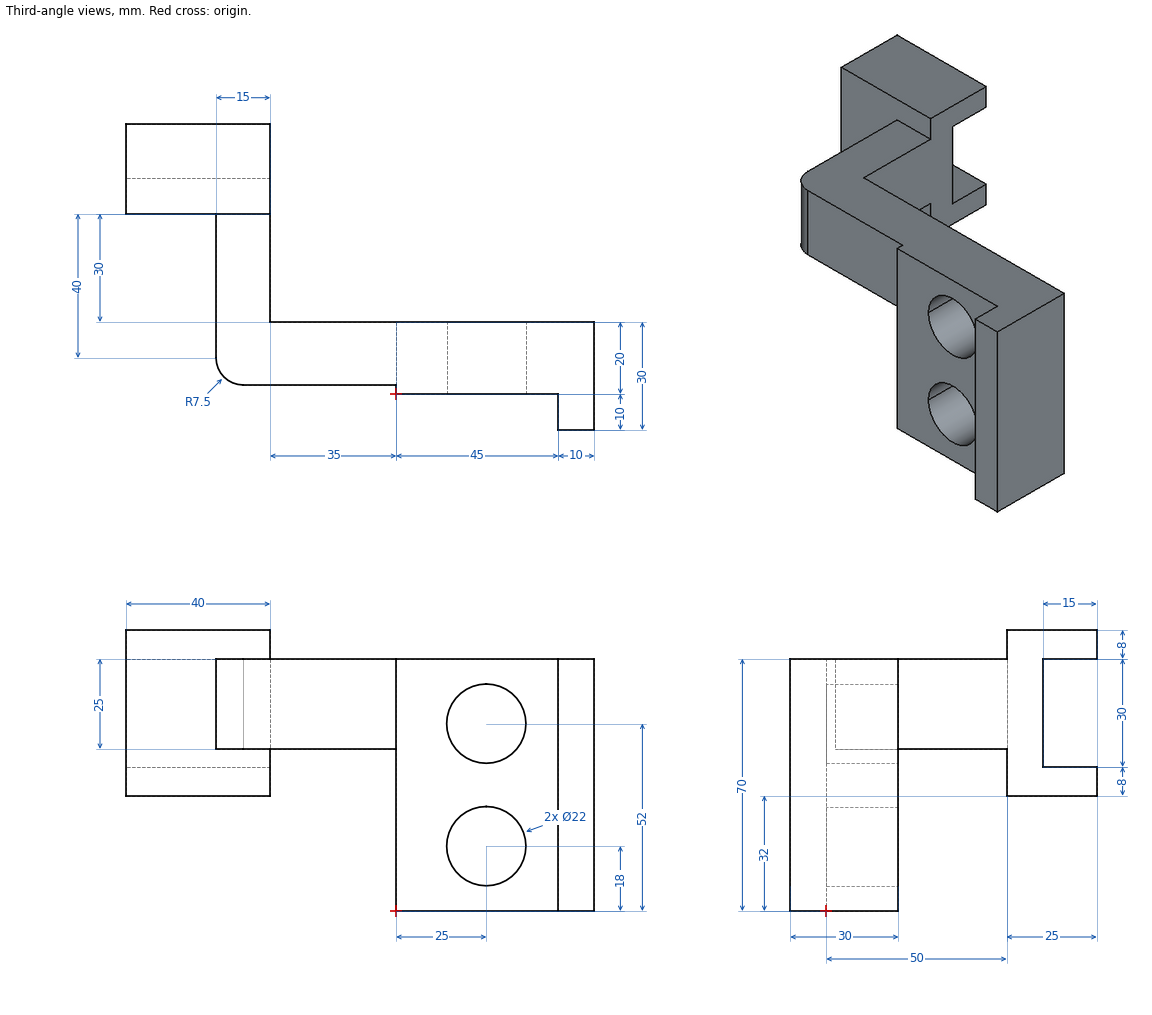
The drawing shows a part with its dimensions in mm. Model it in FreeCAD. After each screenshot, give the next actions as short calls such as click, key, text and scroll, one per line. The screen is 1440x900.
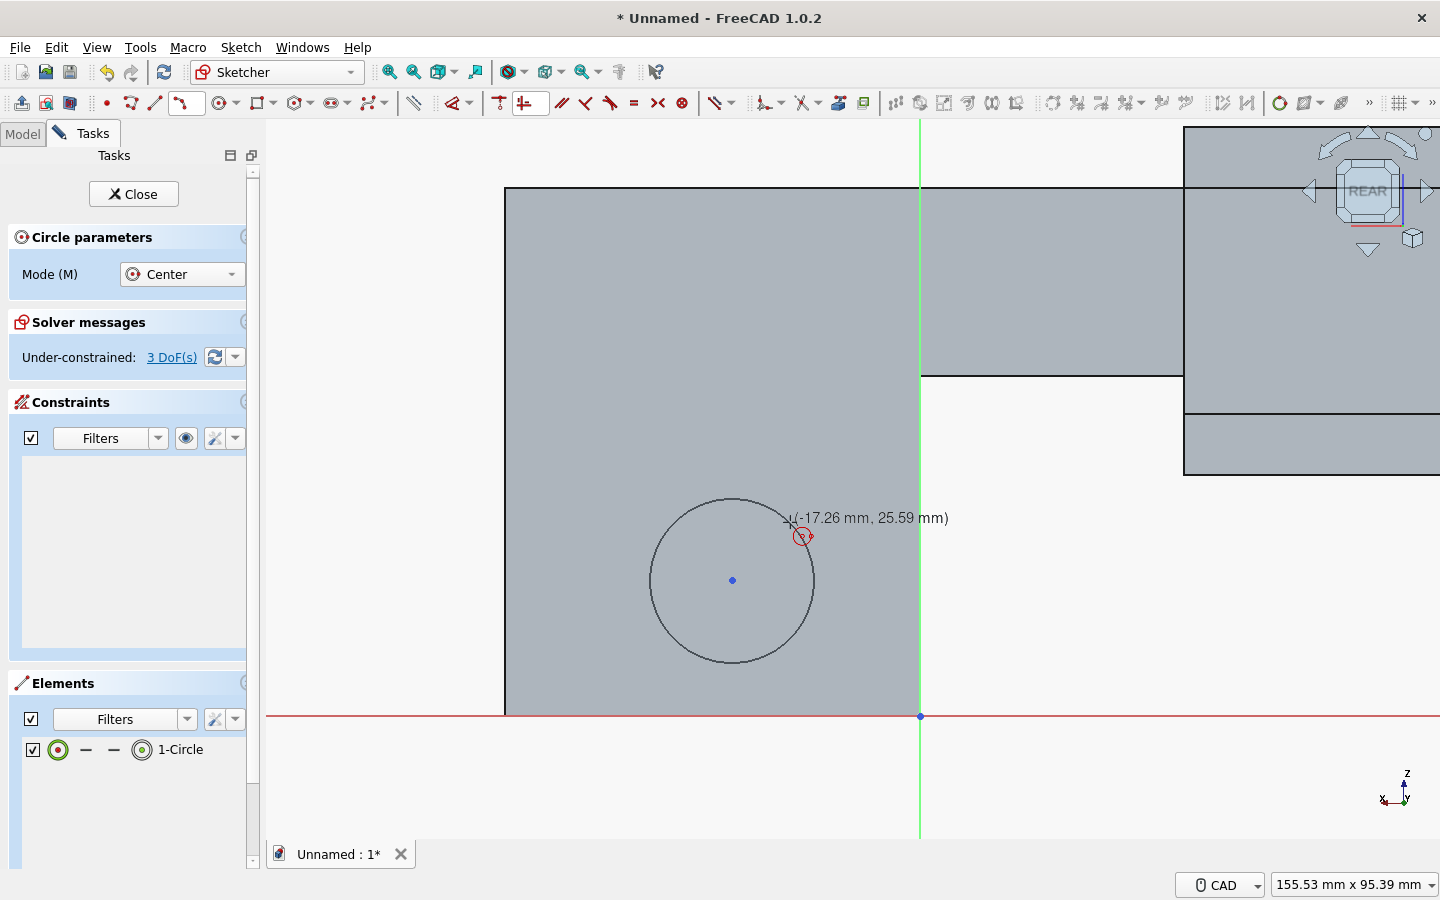
click(732, 324)
click(790, 265)
key(Escape)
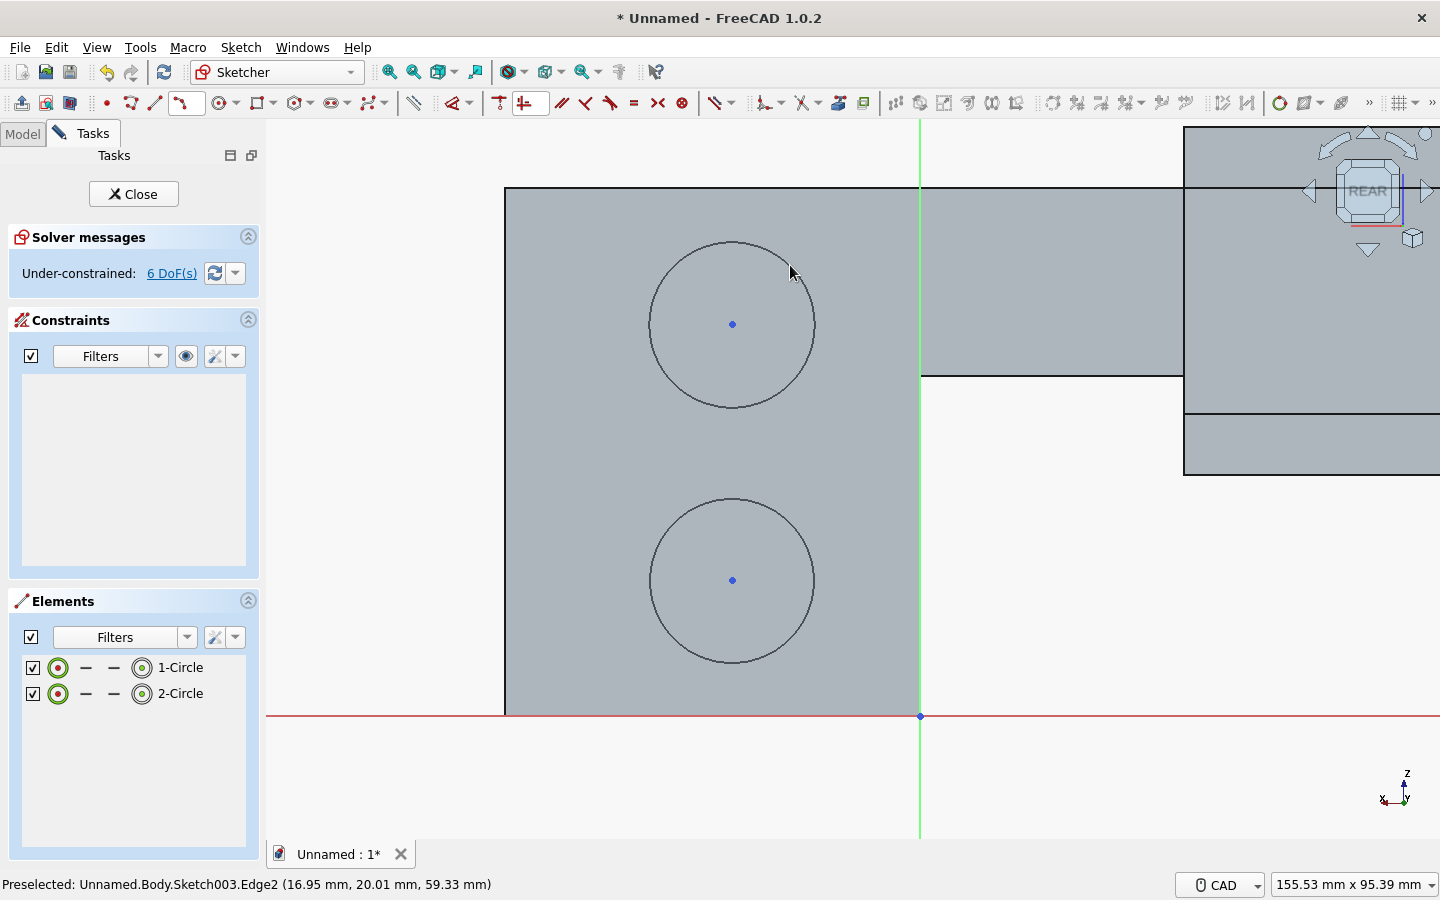
click(790, 523)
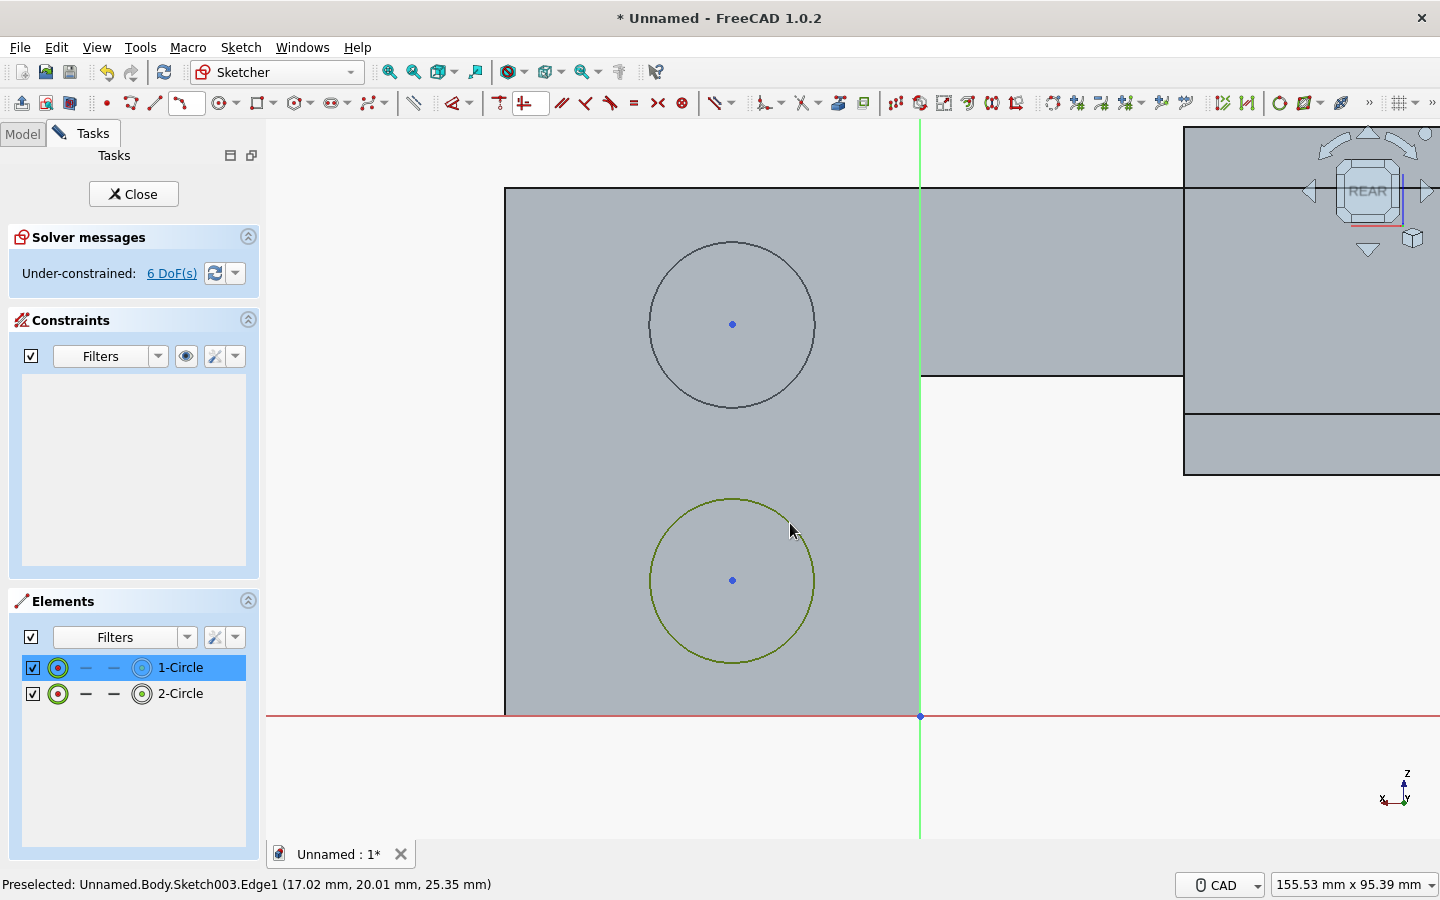
click(790, 266)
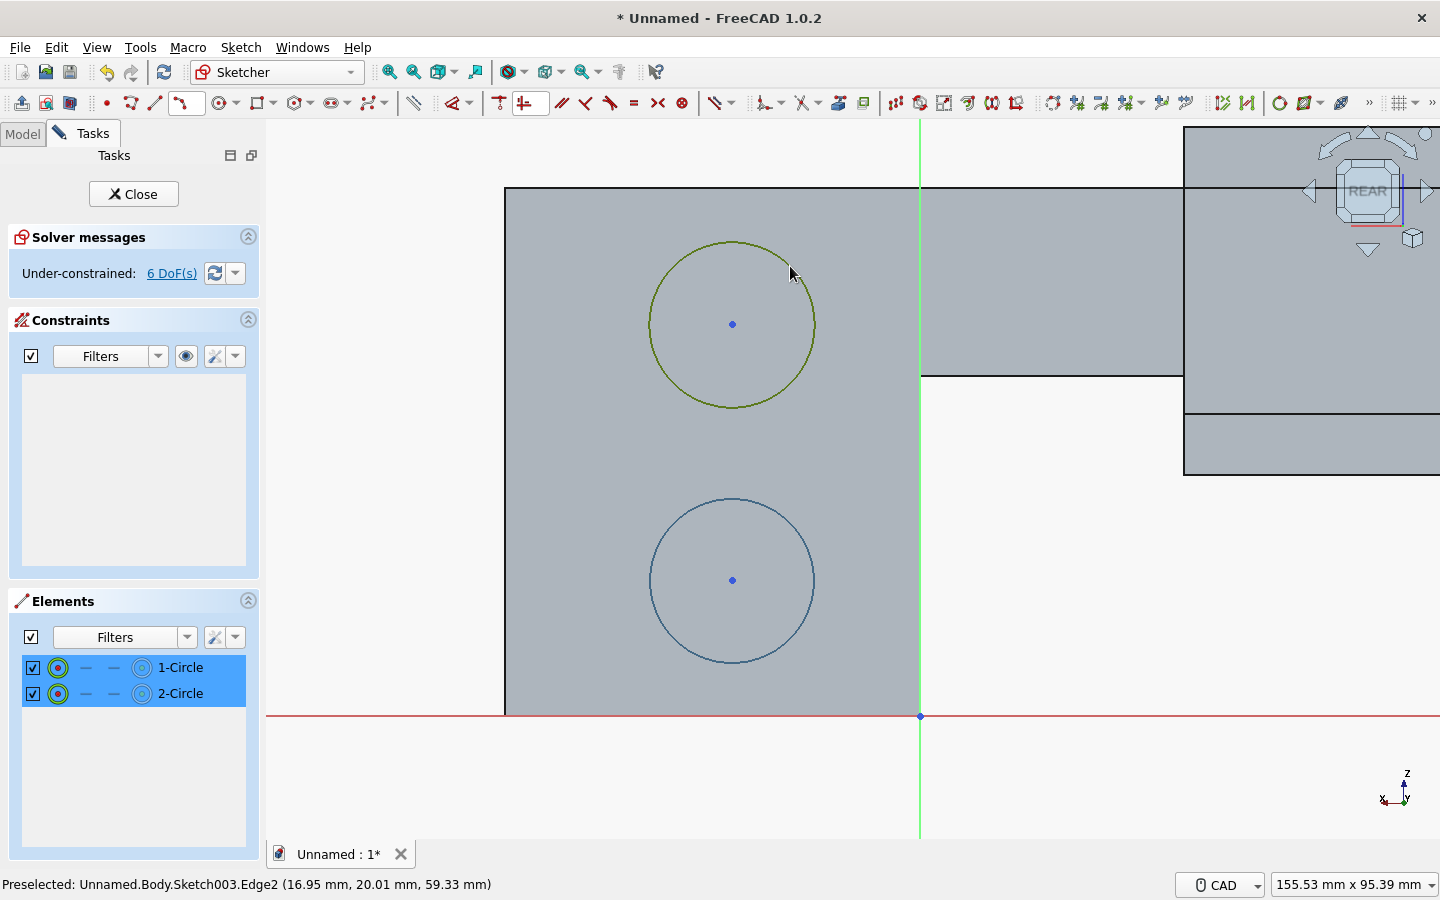
key(e)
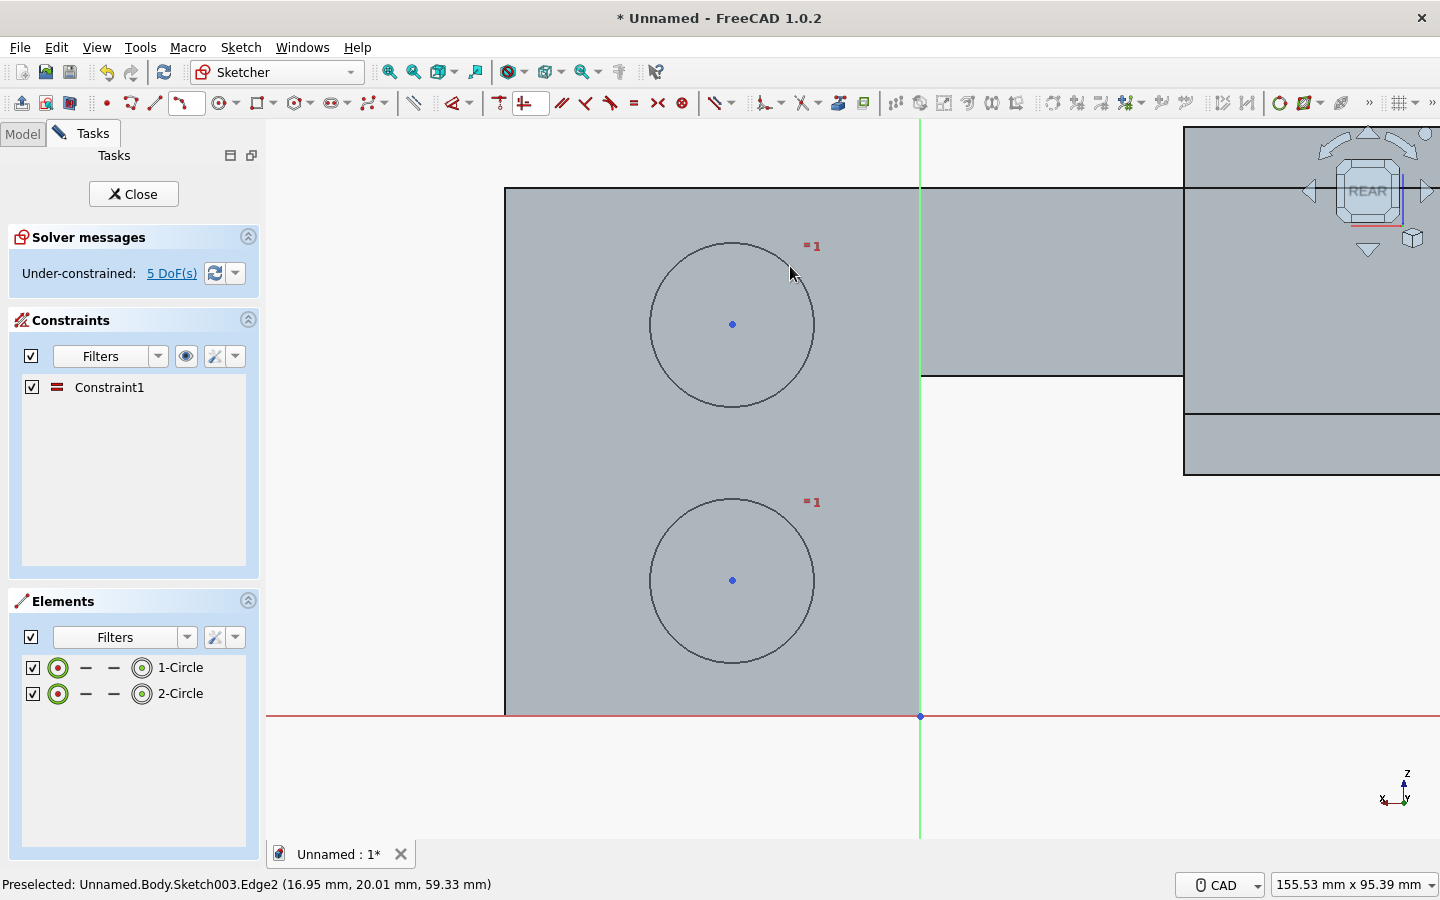
click(732, 581)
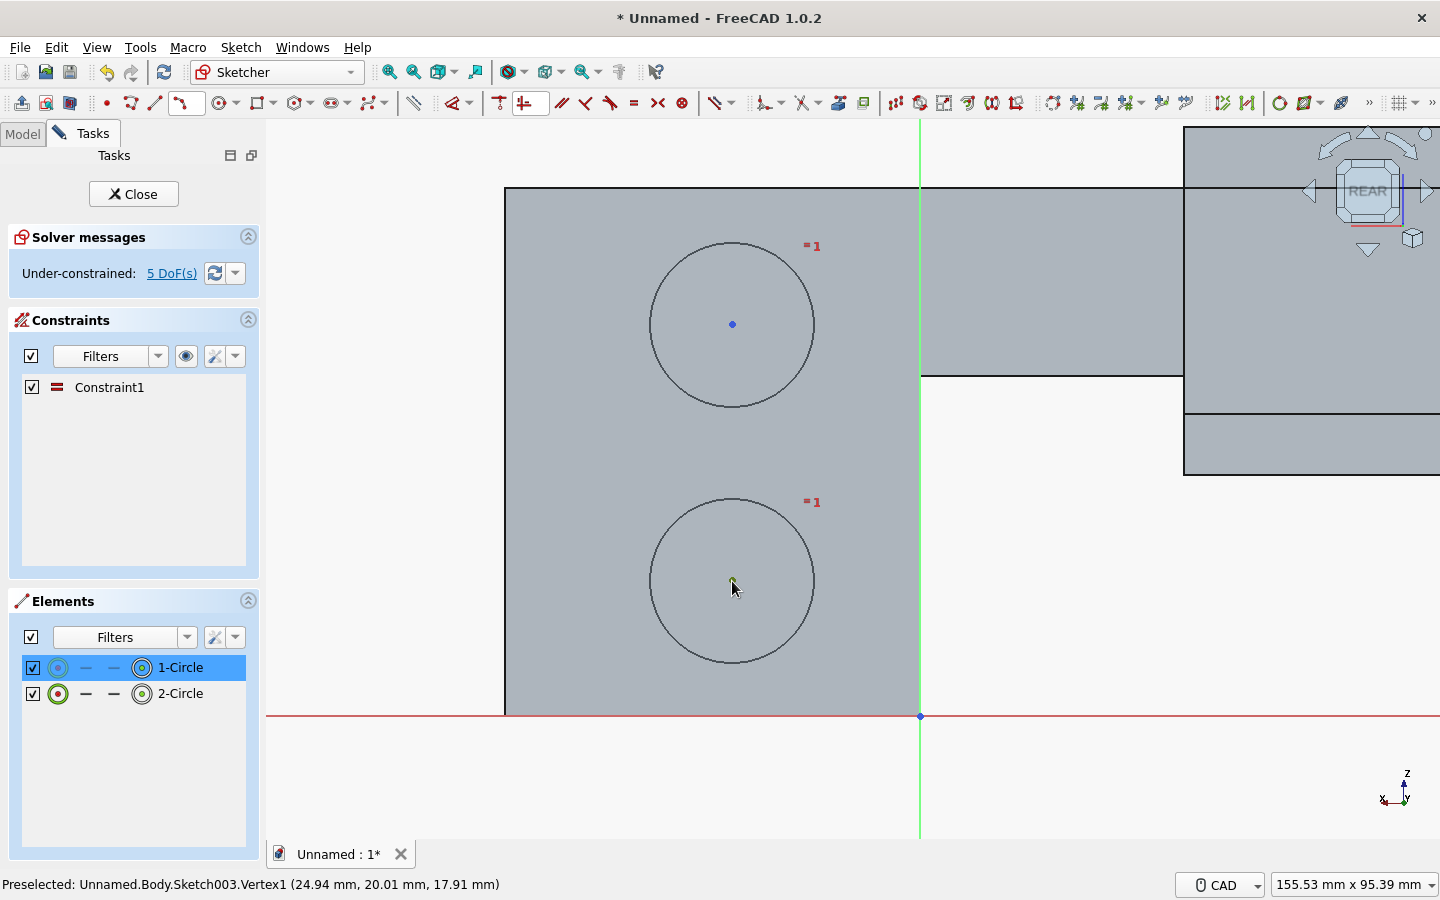
click(732, 325)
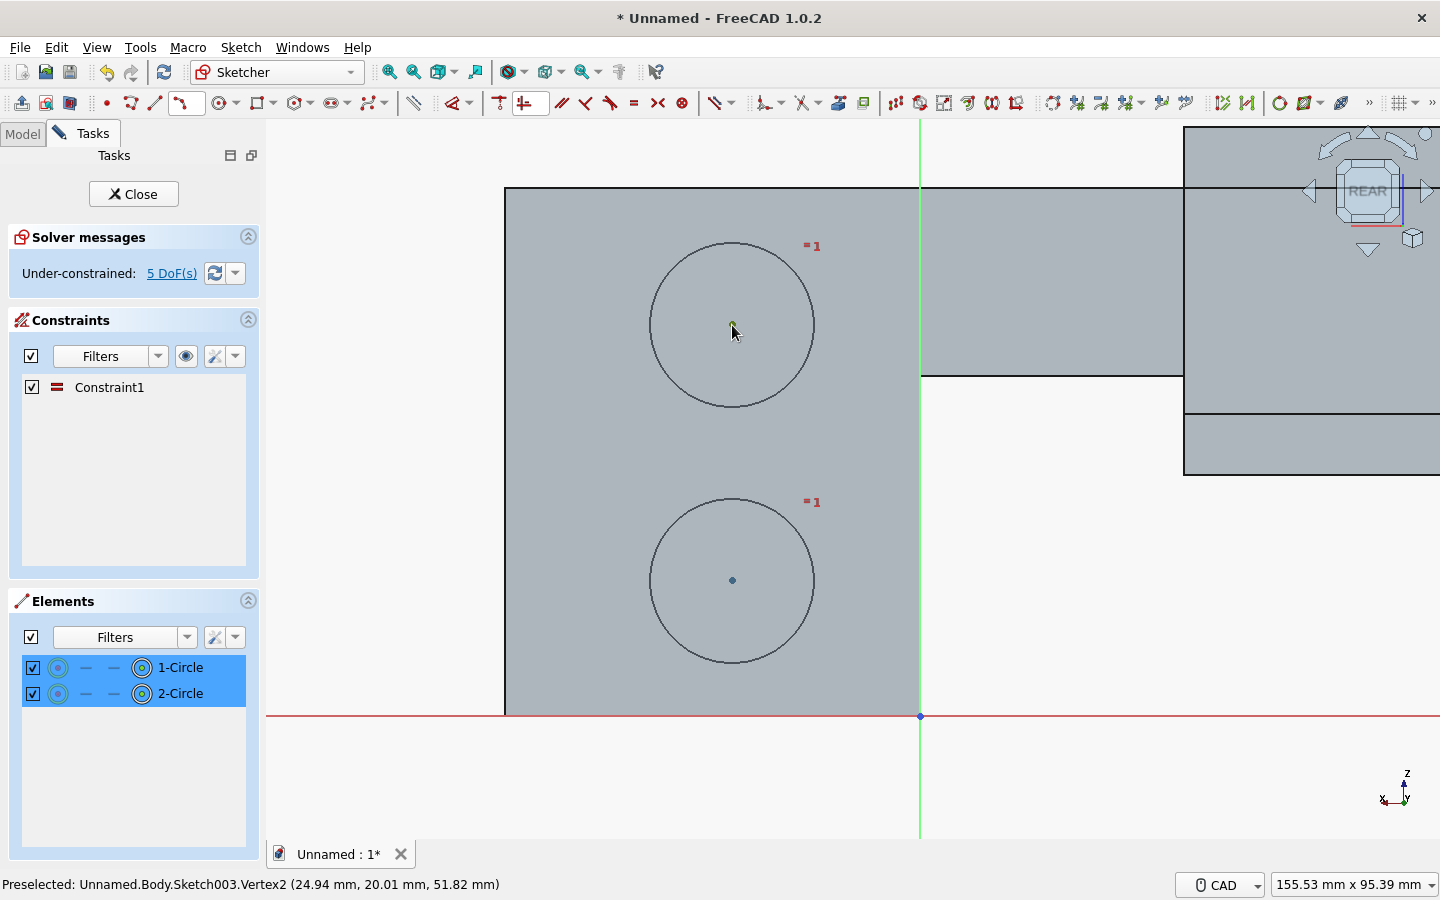
key(v)